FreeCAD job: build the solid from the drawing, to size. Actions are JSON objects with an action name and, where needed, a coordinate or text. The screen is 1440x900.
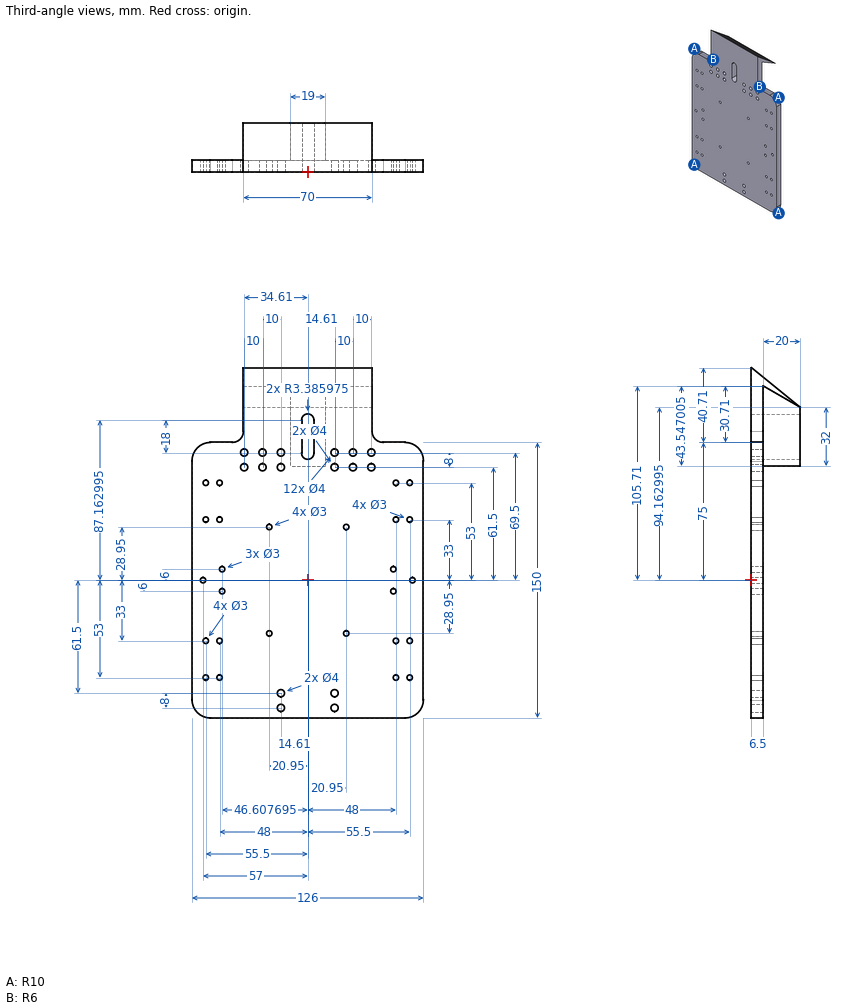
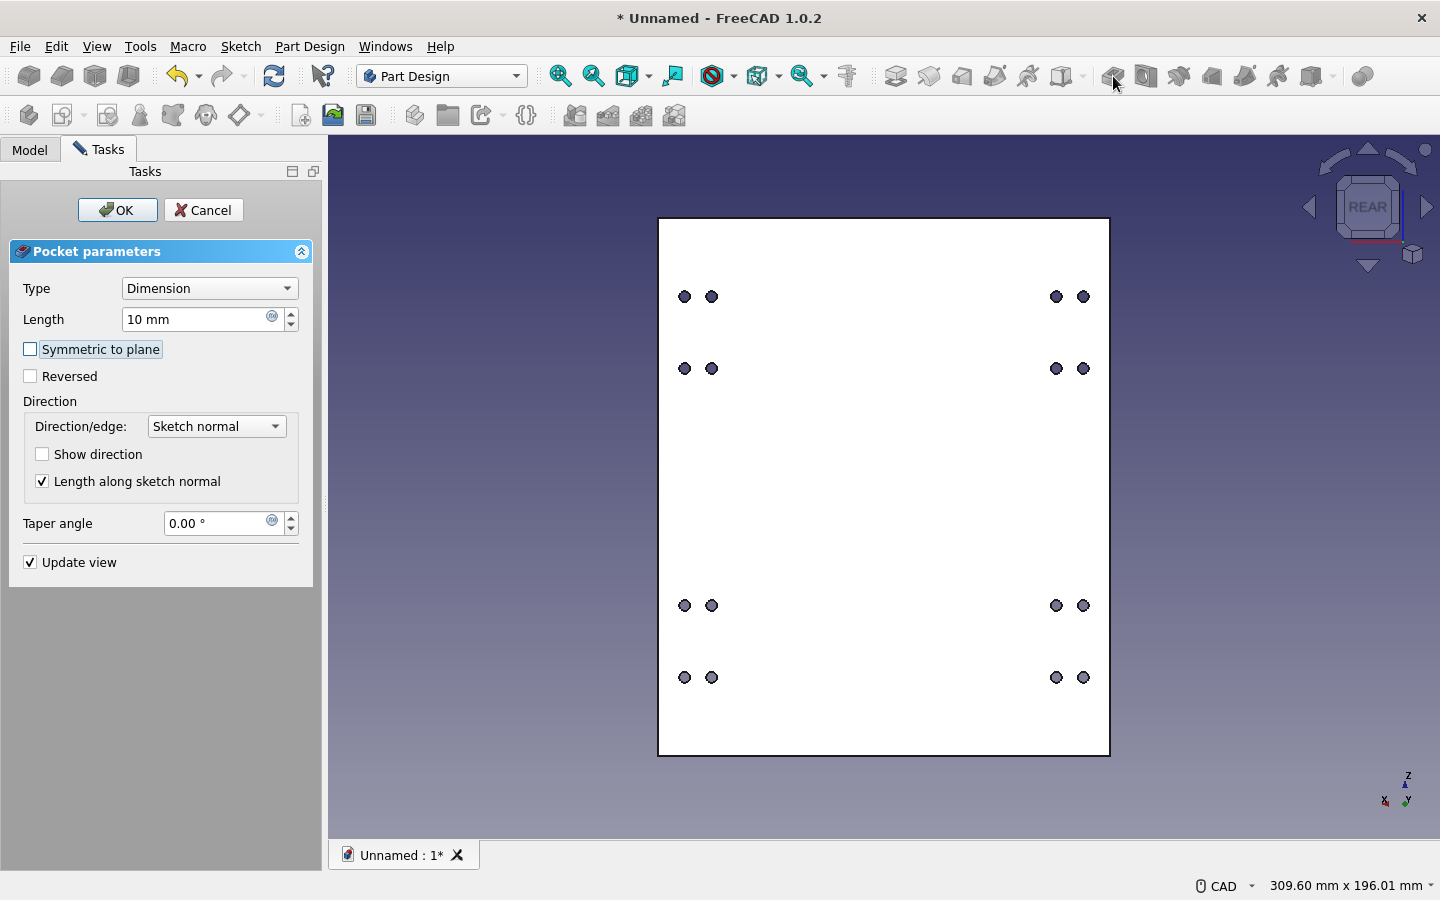
{"action": "left_click", "coordinate": [118, 210]}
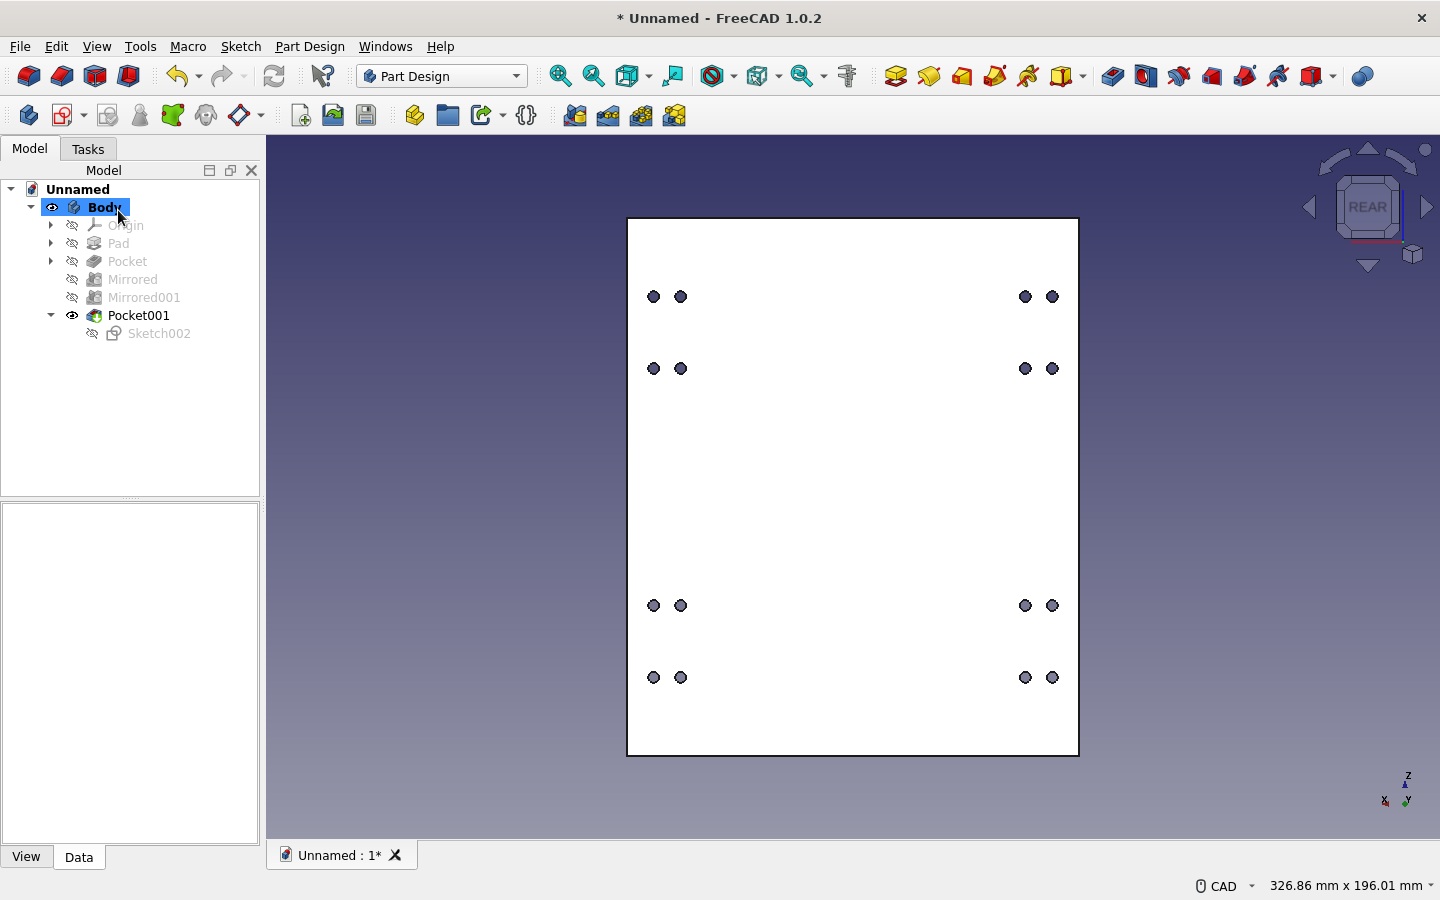
{"action": "left_click", "coordinate": [853, 486]}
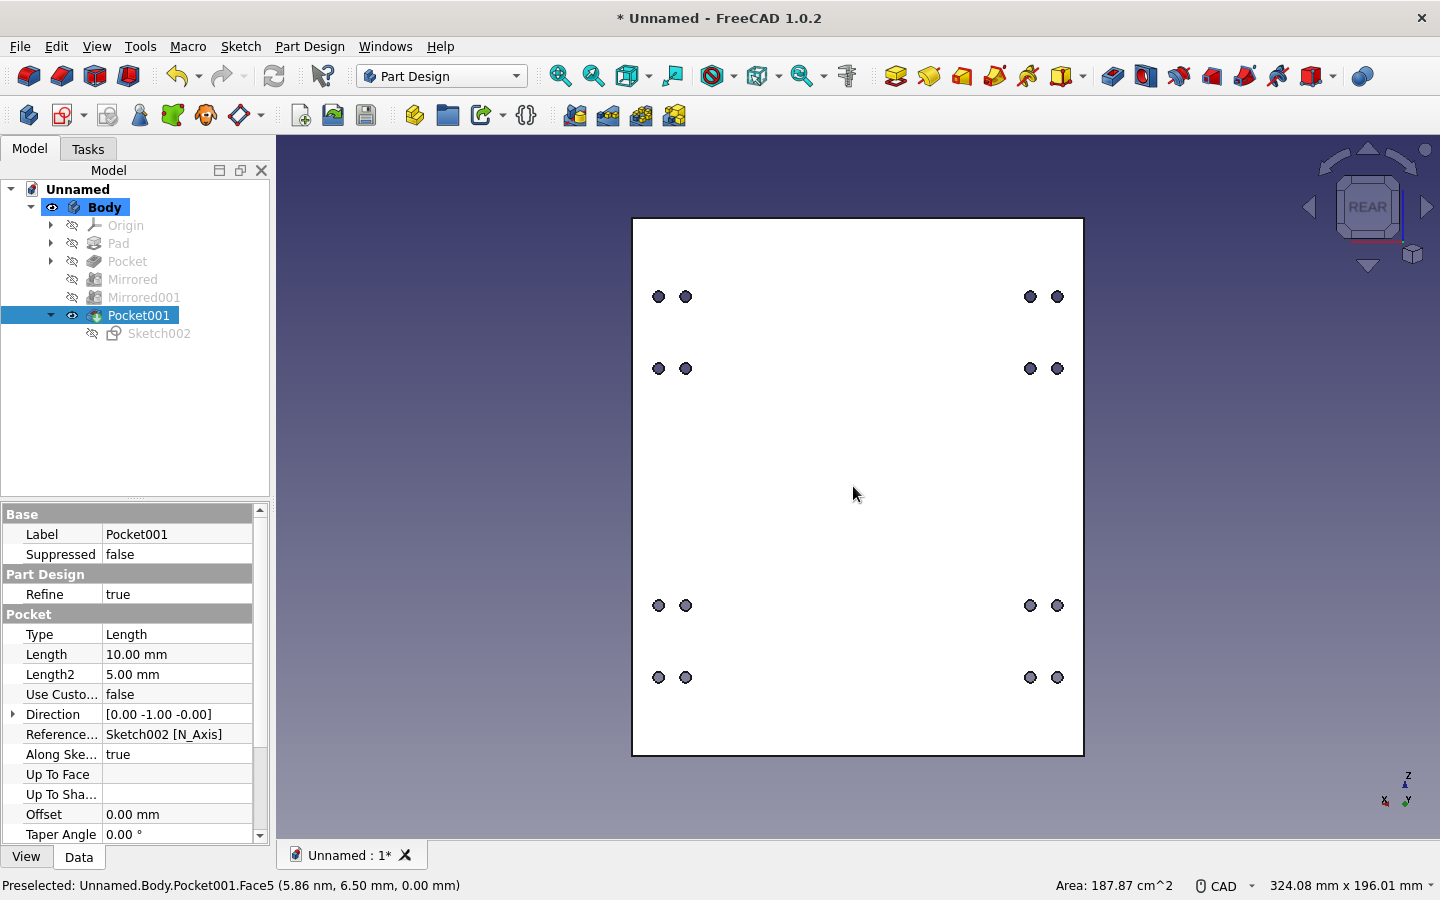
{"action": "left_click", "coordinate": [62, 116]}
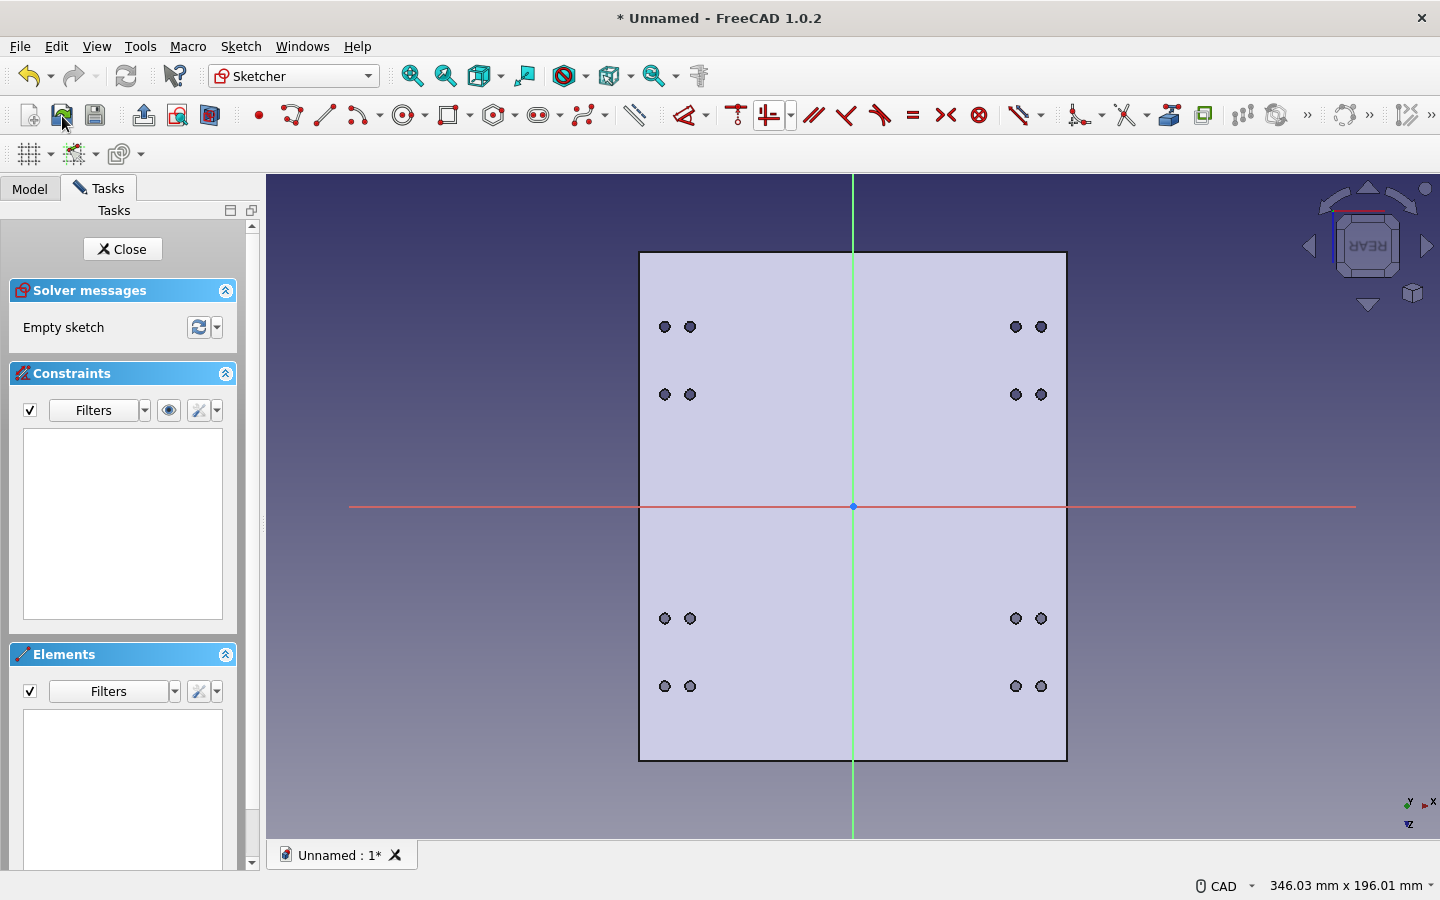
{"action": "scroll", "coordinate": [909, 506], "scroll_direction": "up", "scroll_amount": 4}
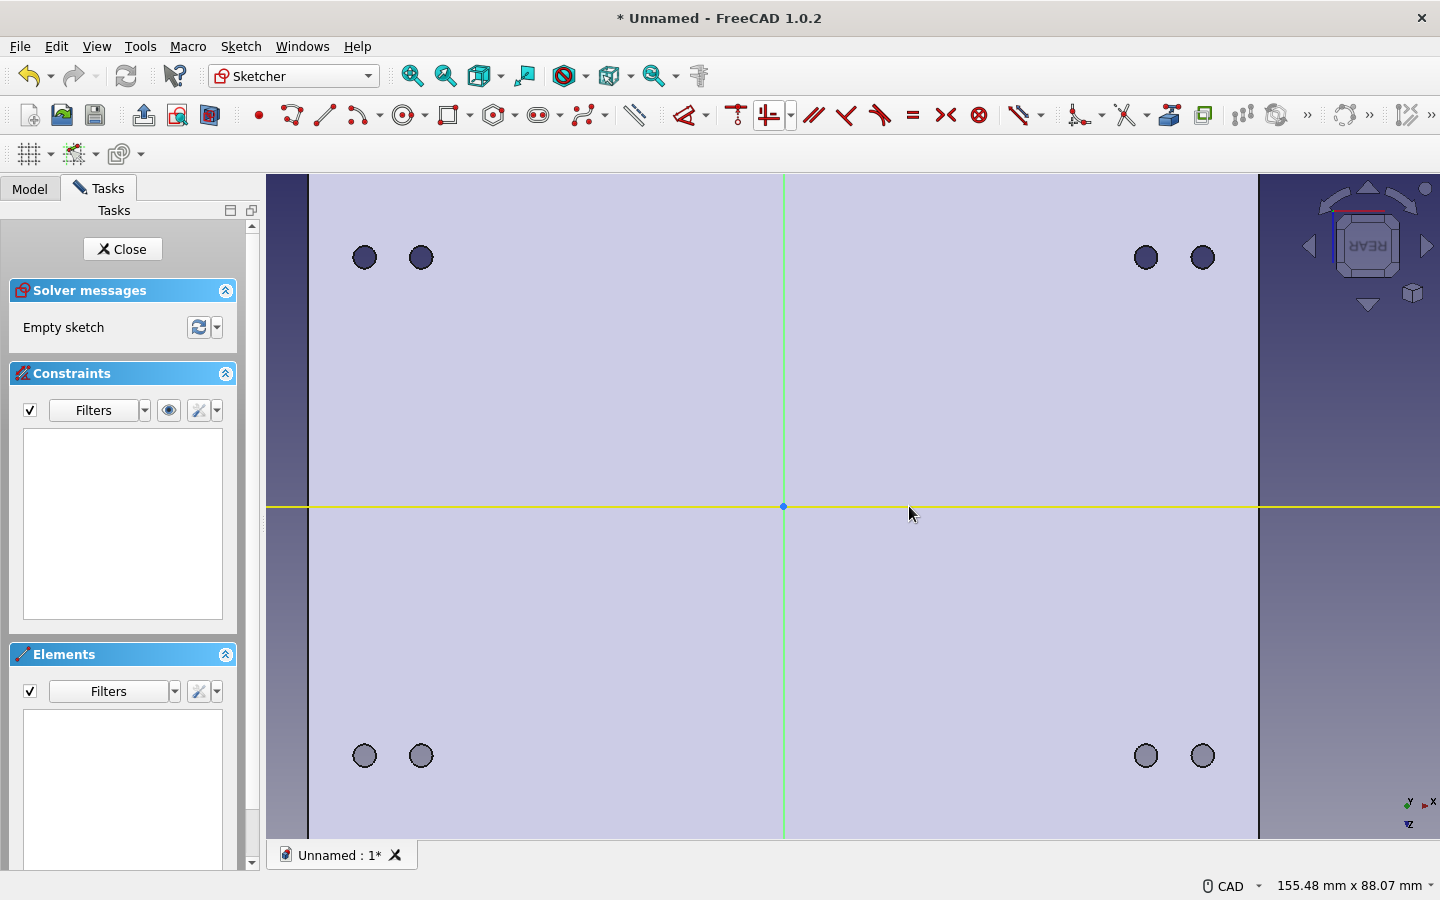
{"action": "left_click", "coordinate": [402, 116]}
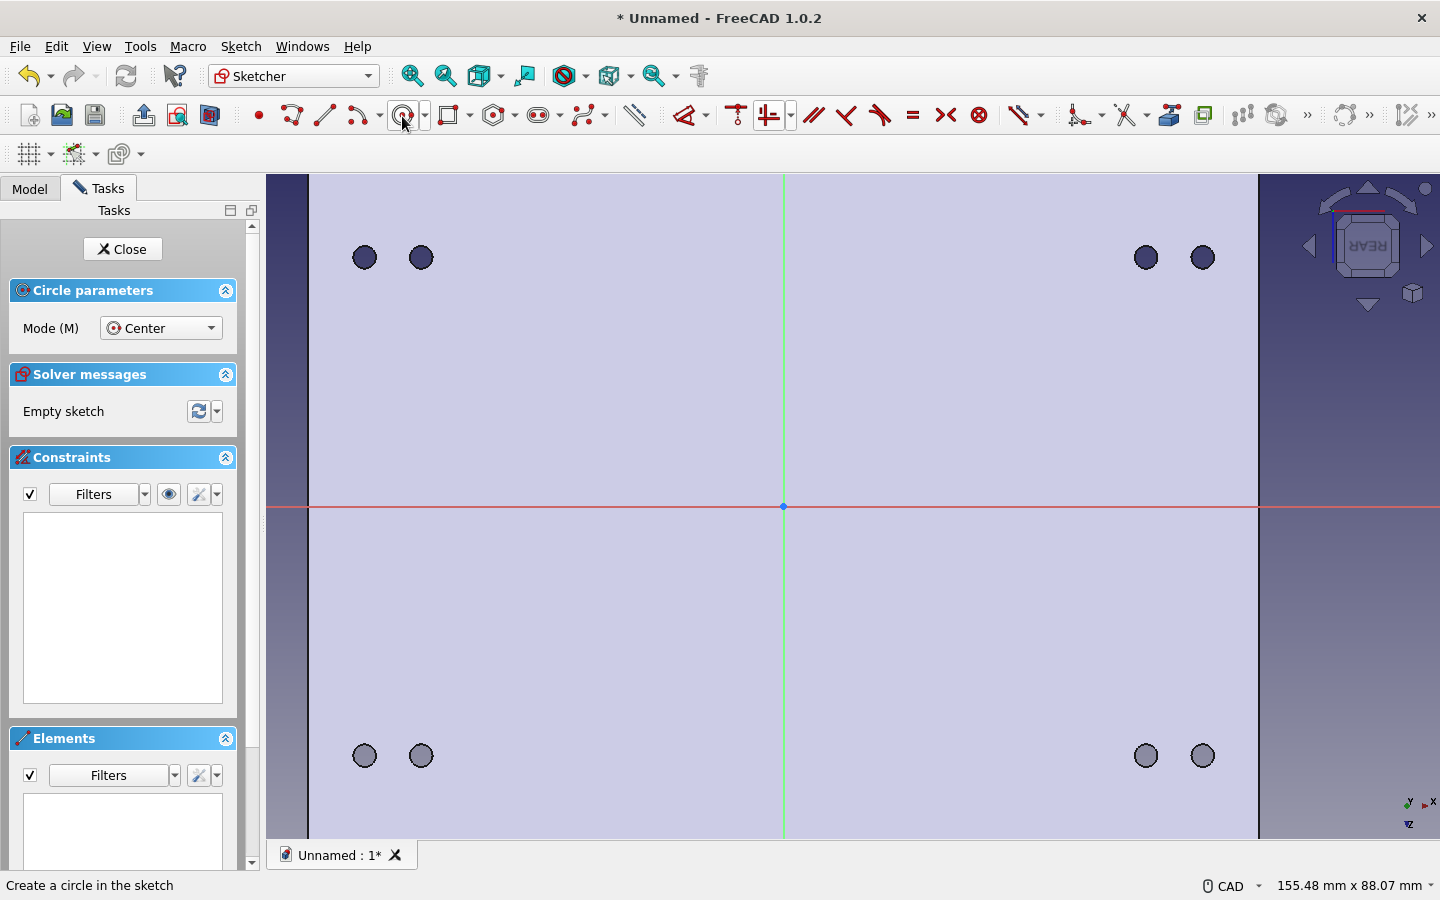
{"action": "scroll", "coordinate": [626, 725], "scroll_direction": "up", "scroll_amount": 4}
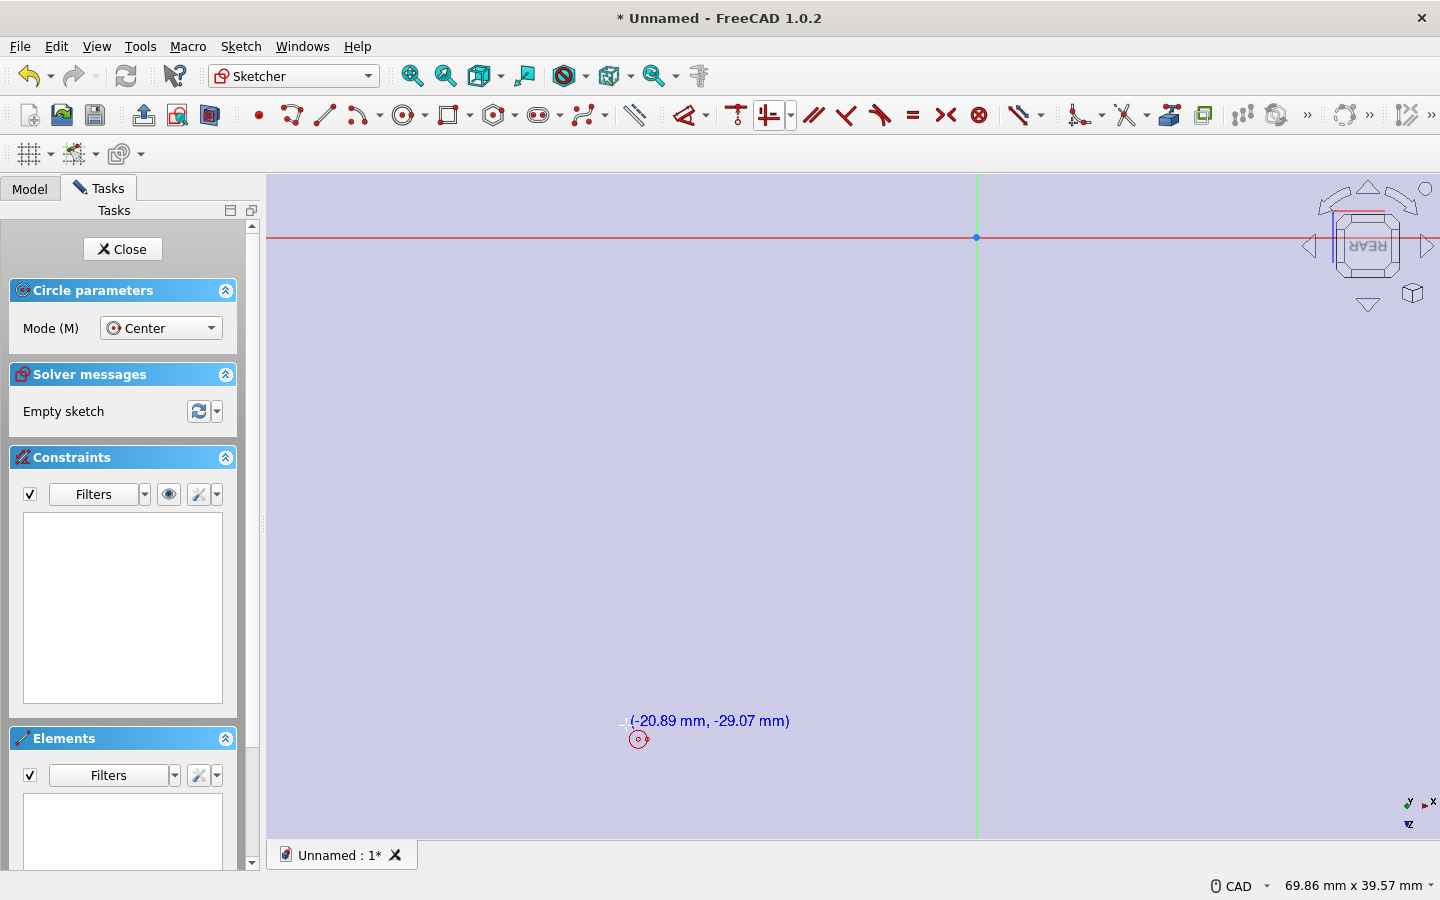
{"action": "left_click", "coordinate": [625, 724]}
{"action": "mouse_move", "coordinate": [642, 706]}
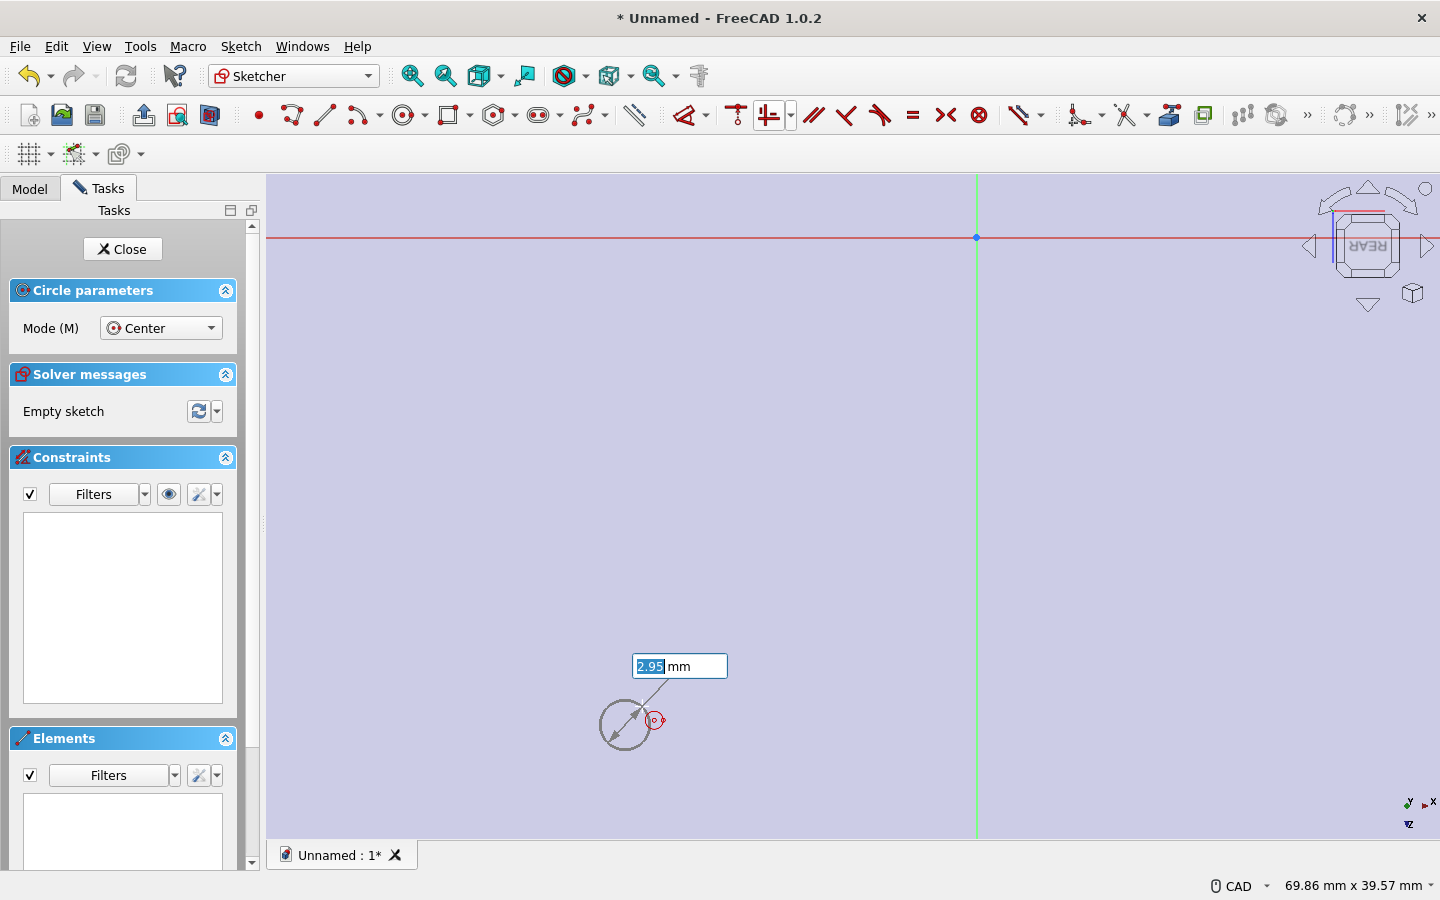
{"action": "type", "text": "3"}
{"action": "key", "text": "Return"}